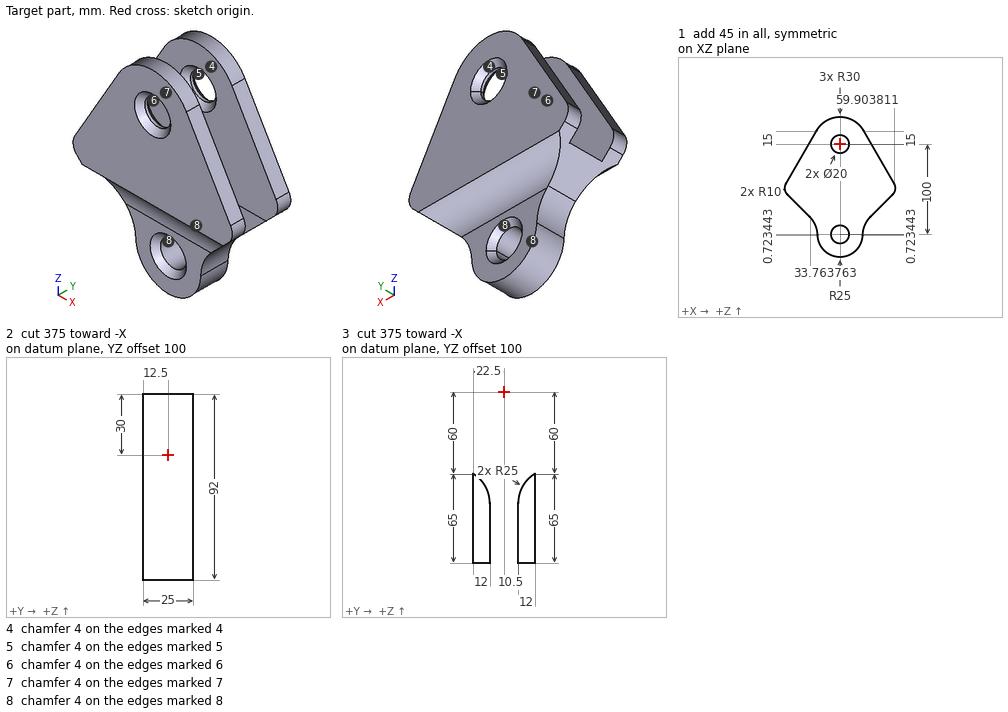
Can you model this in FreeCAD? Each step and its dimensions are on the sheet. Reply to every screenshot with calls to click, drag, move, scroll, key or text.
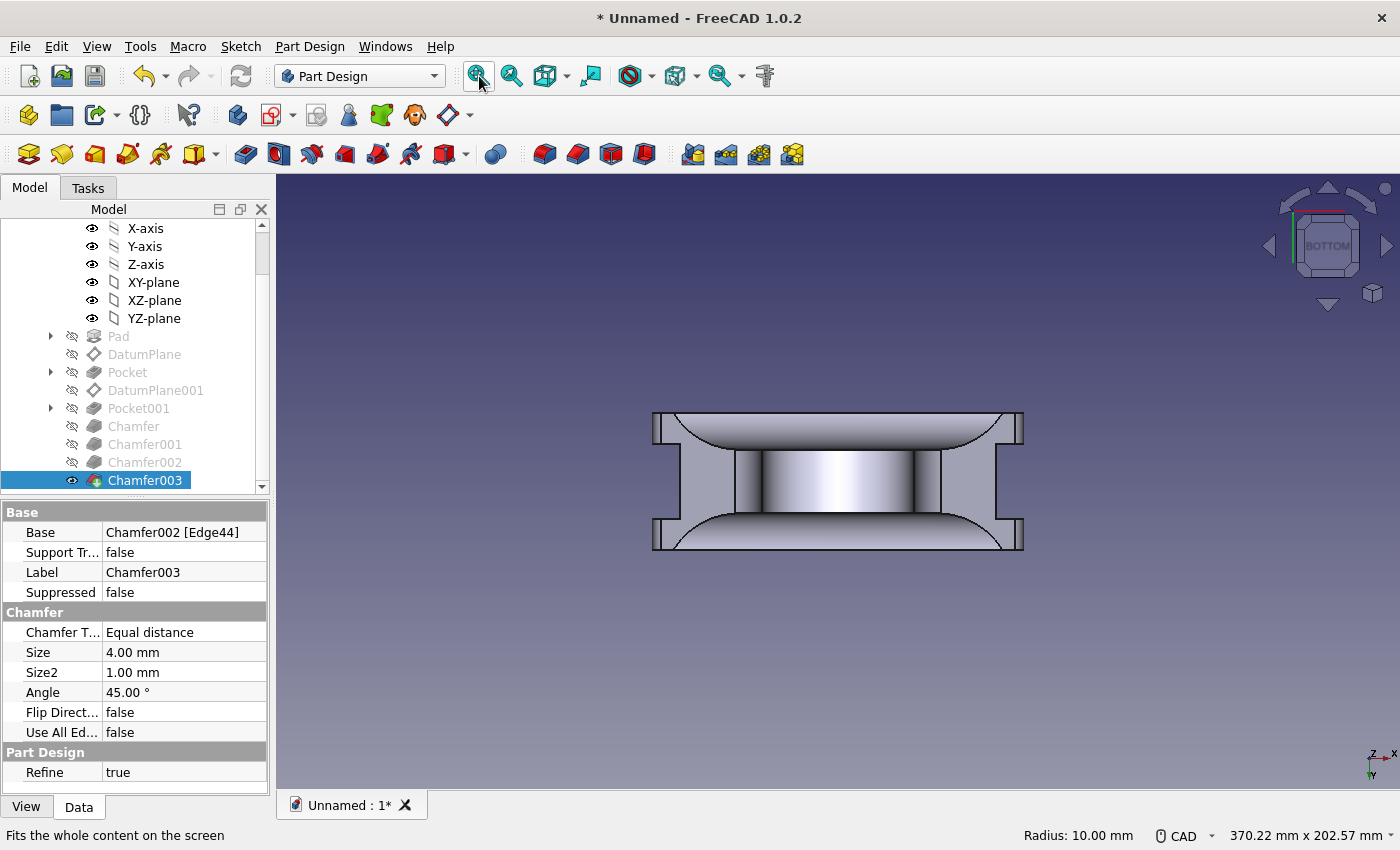
click(479, 76)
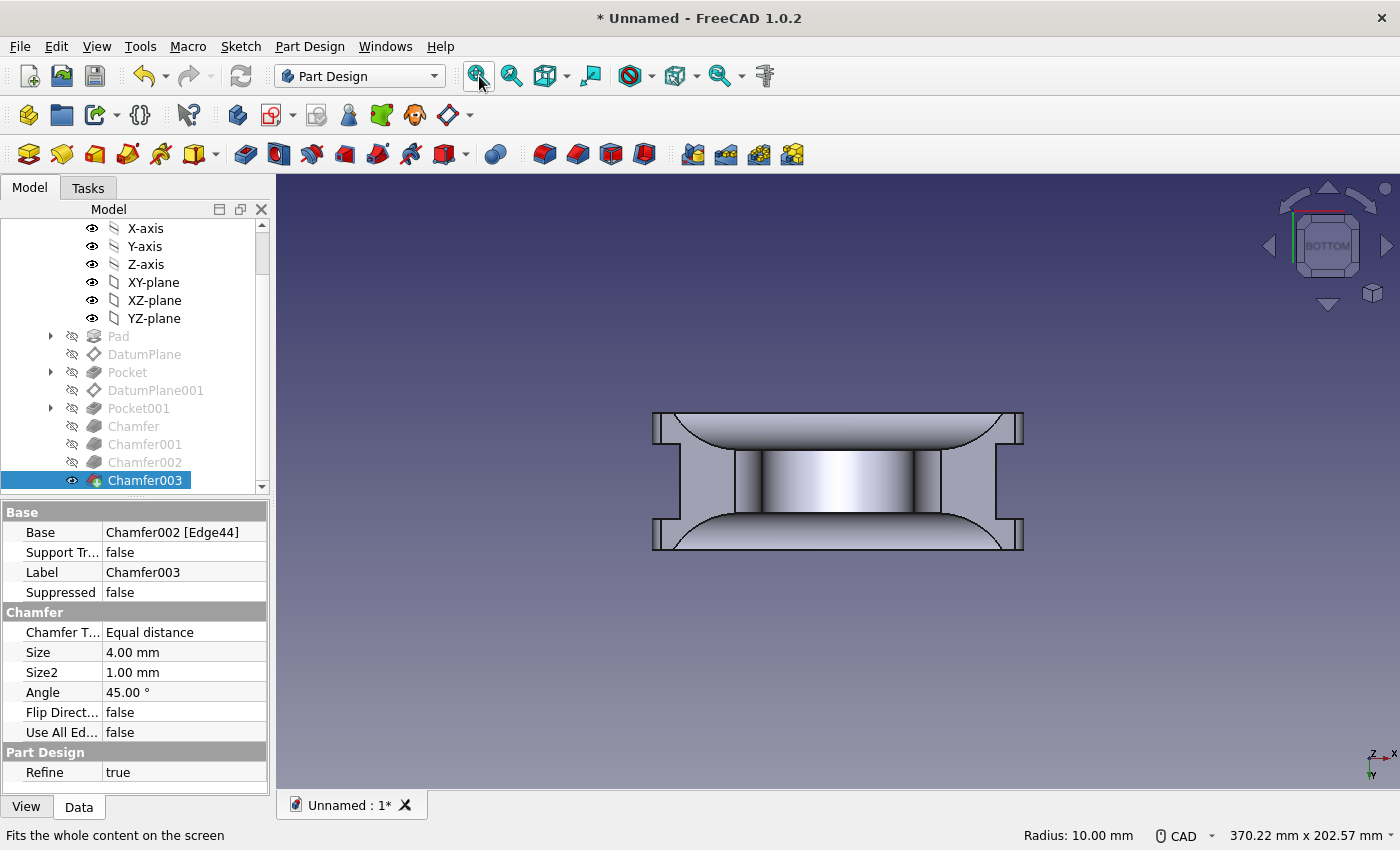
key(4)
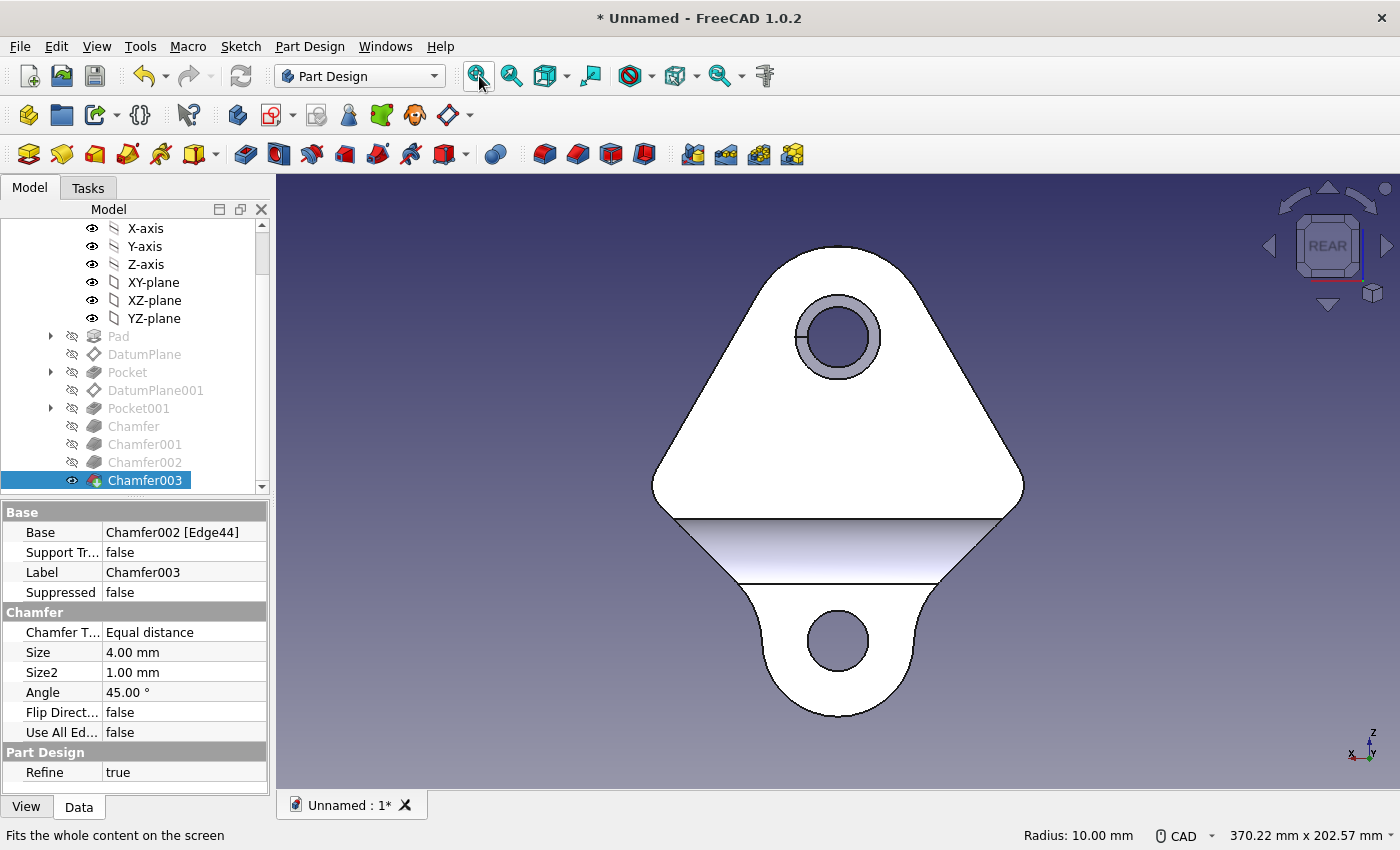
click(863, 658, ctrl)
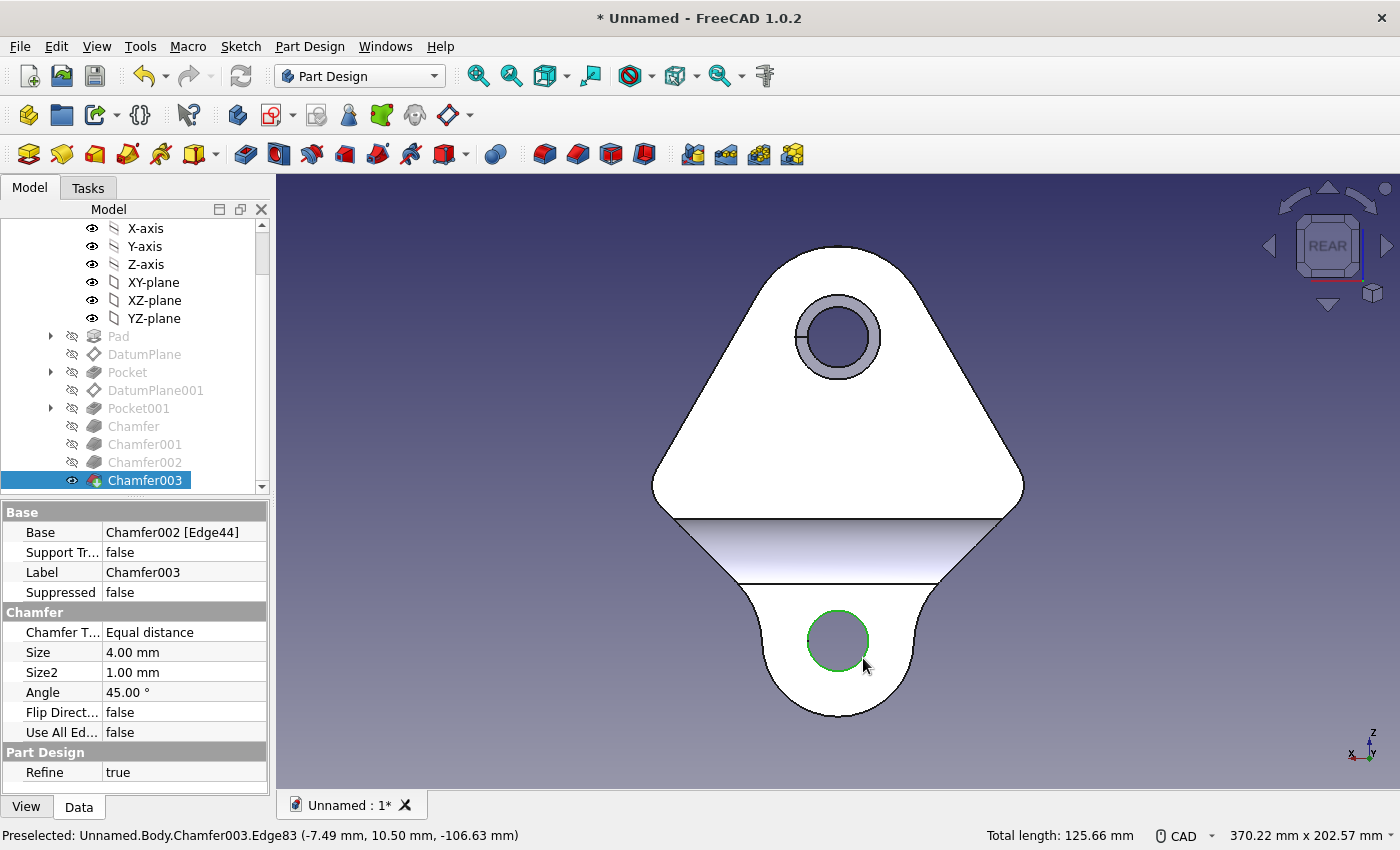
click(578, 154)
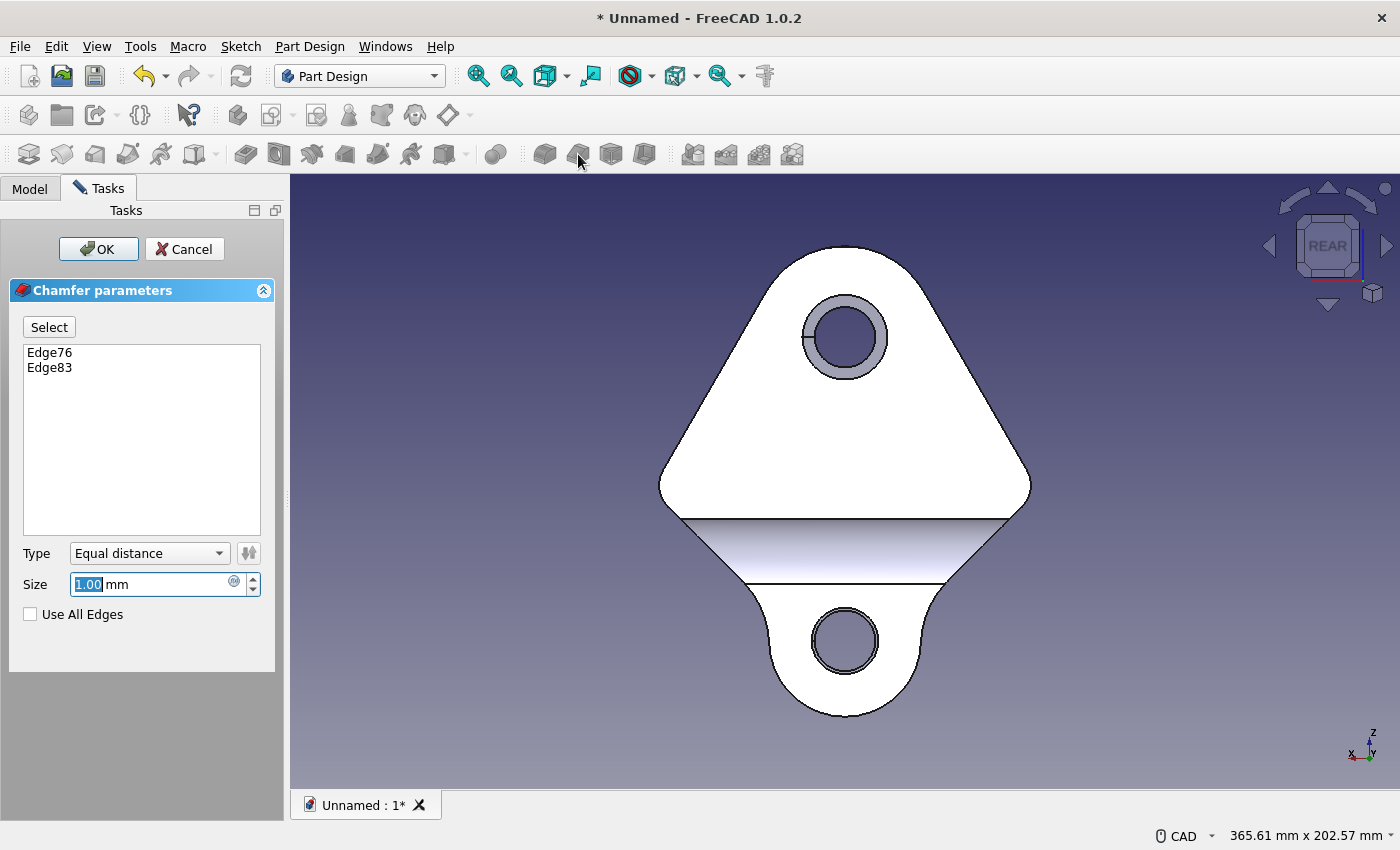
text(4)
key(Tab)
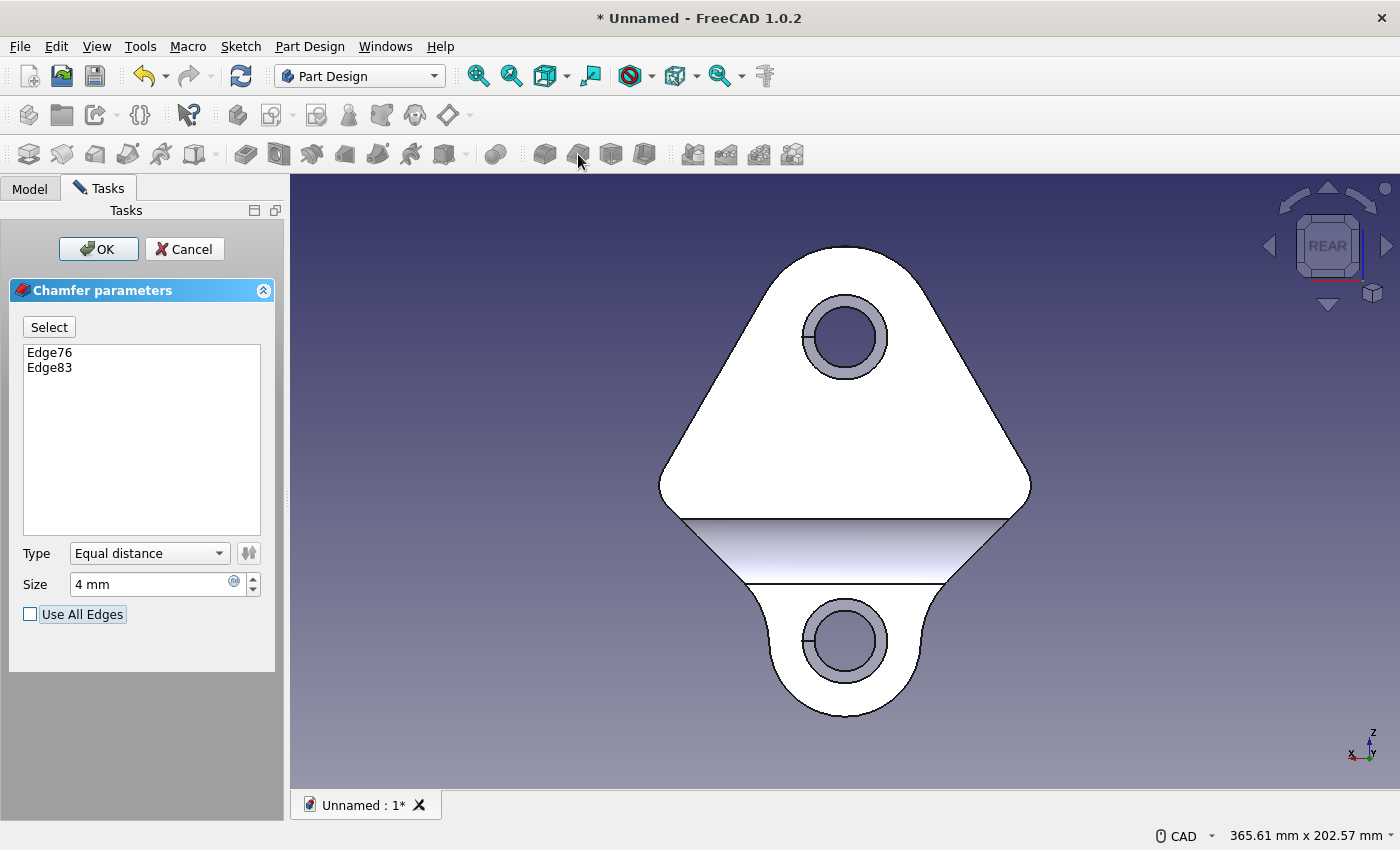
click(99, 249)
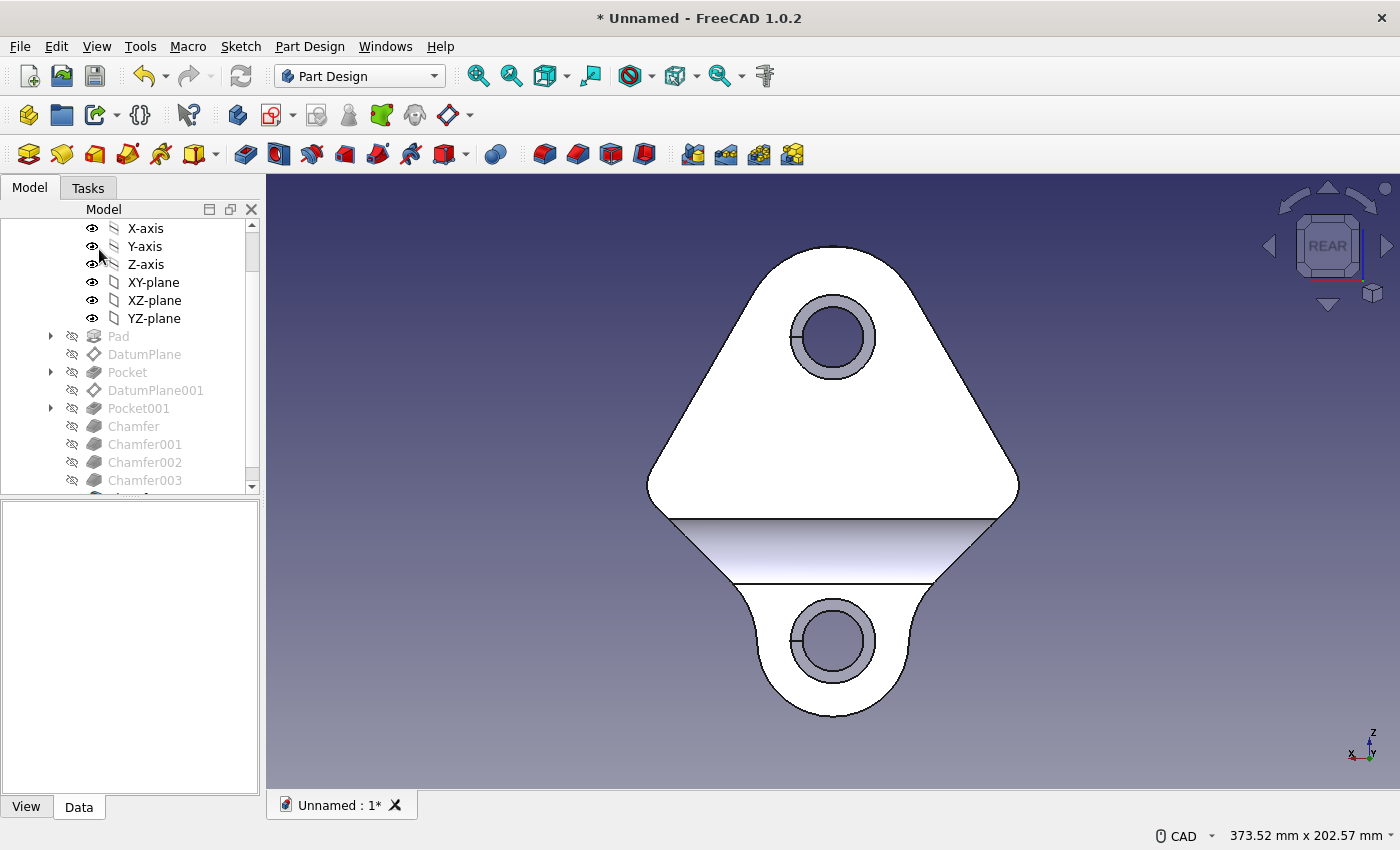
key(0)